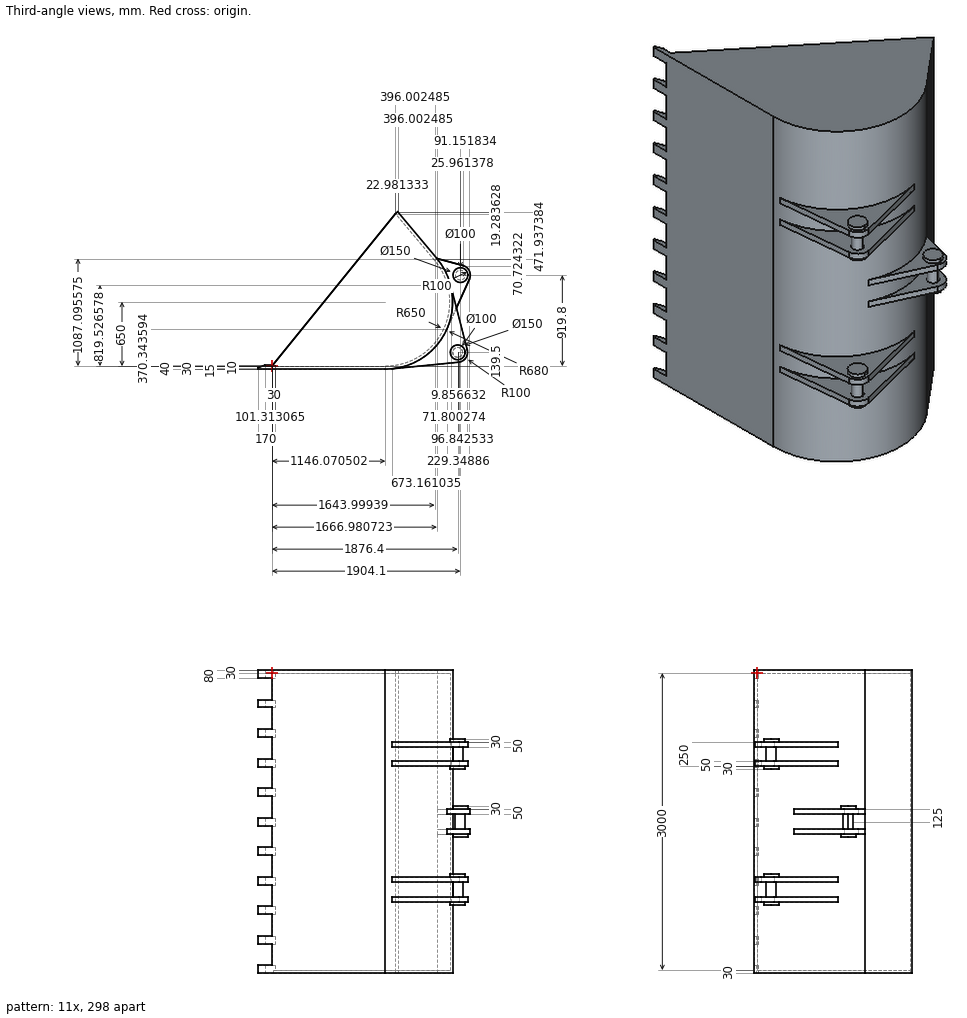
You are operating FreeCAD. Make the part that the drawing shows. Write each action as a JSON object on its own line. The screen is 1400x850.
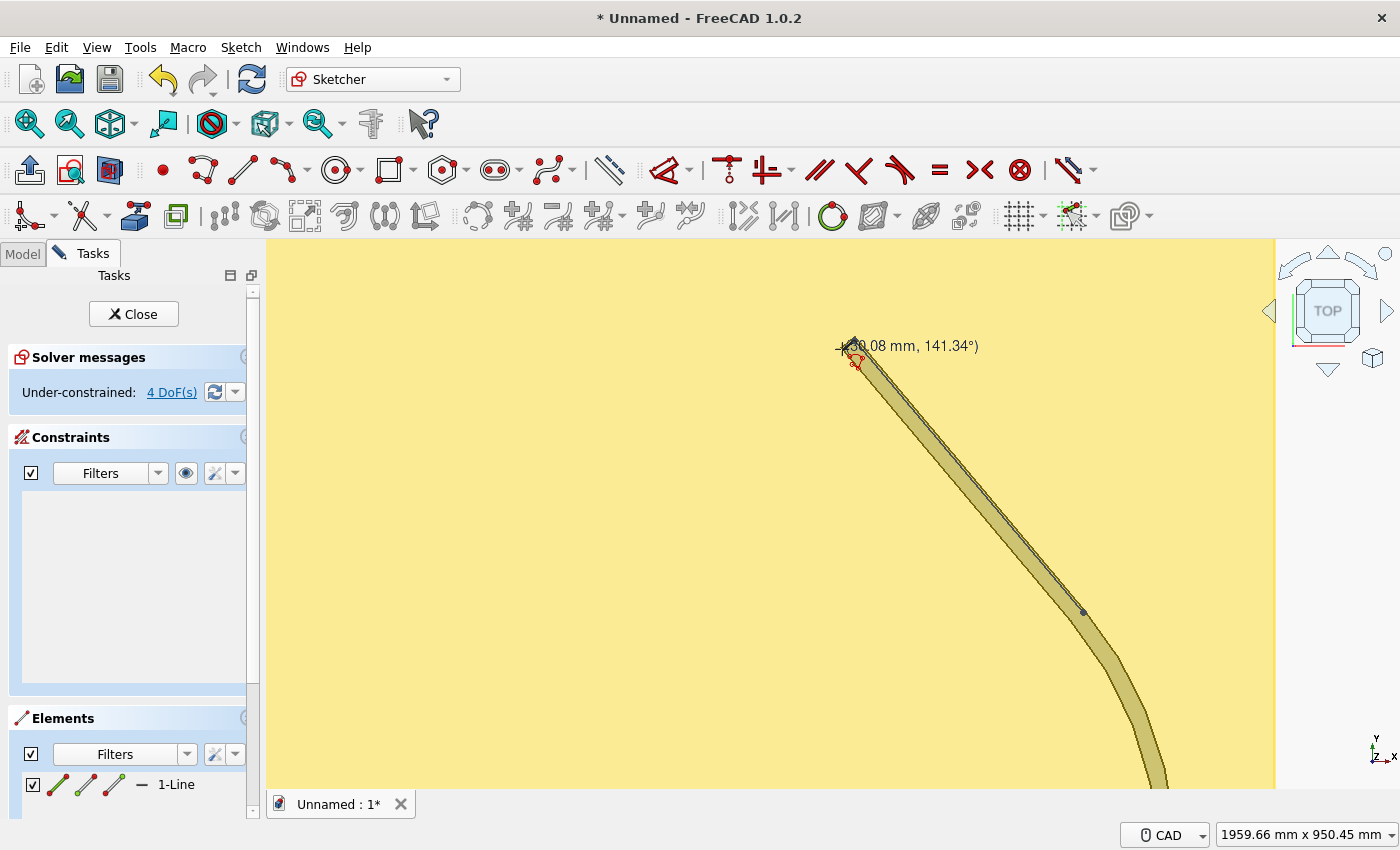
{"action": "left_click", "coordinate": [842, 348]}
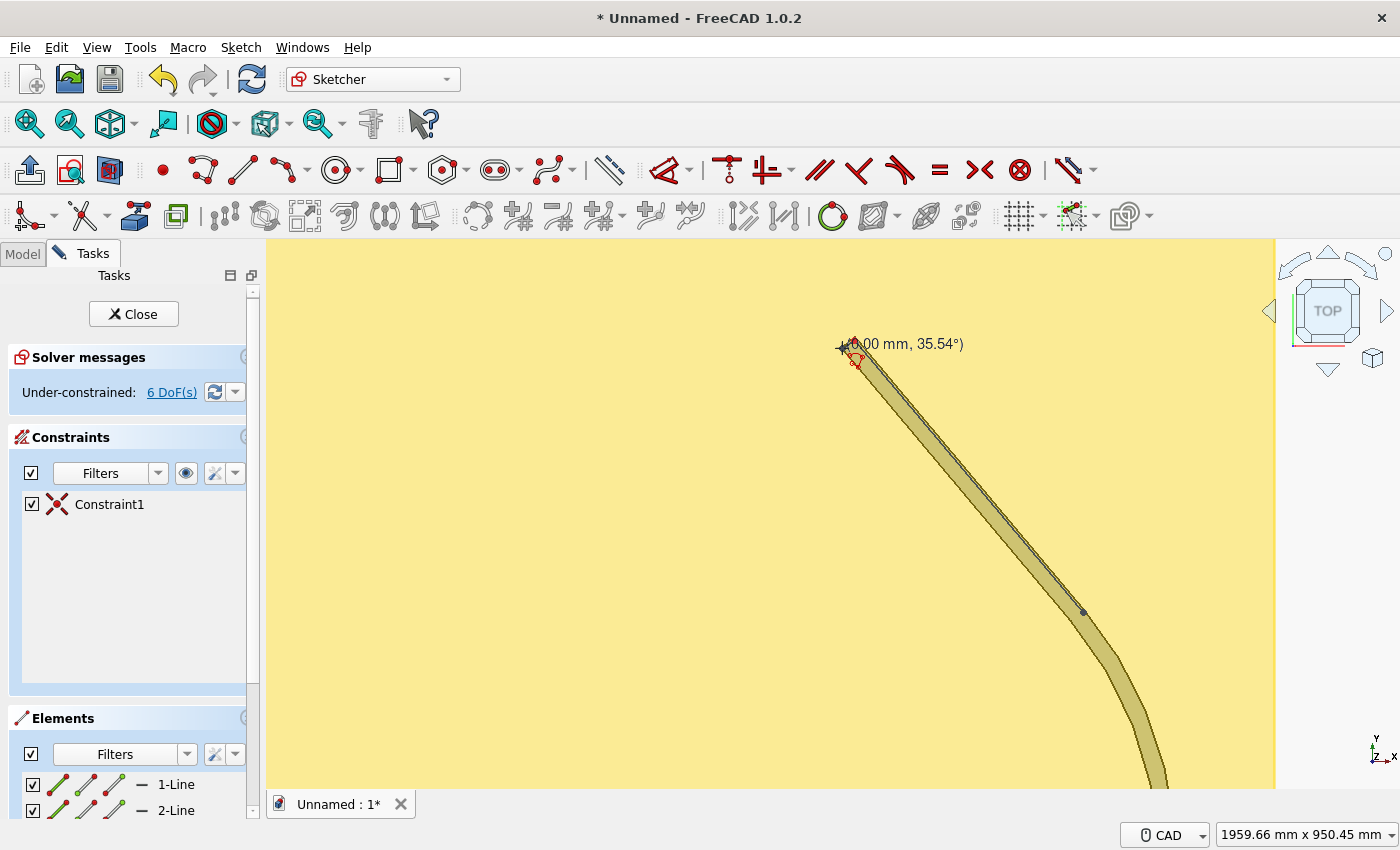
{"action": "scroll", "coordinate": [843, 350], "scroll_direction": "down", "scroll_amount": 5}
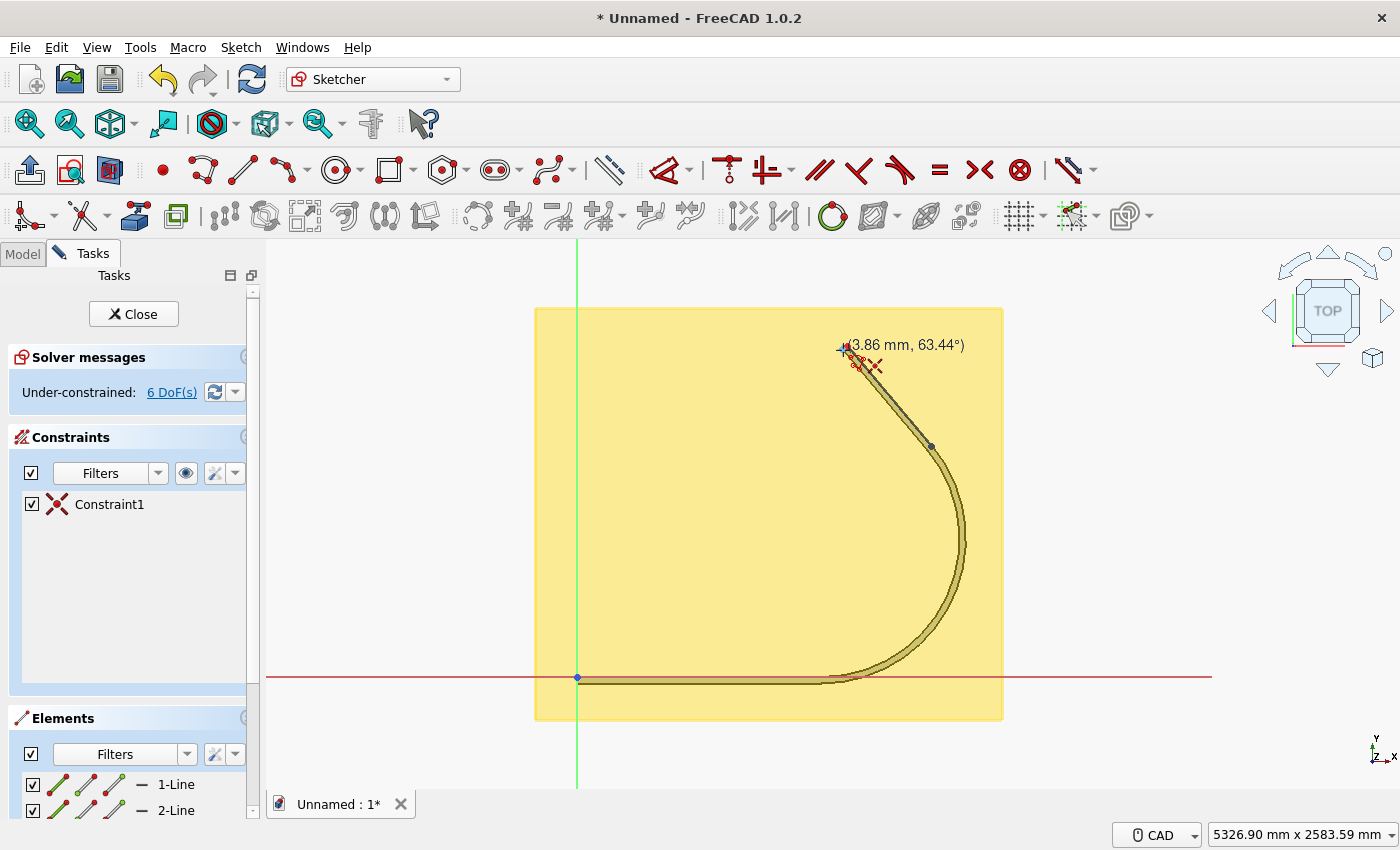
{"action": "left_click", "coordinate": [577, 677]}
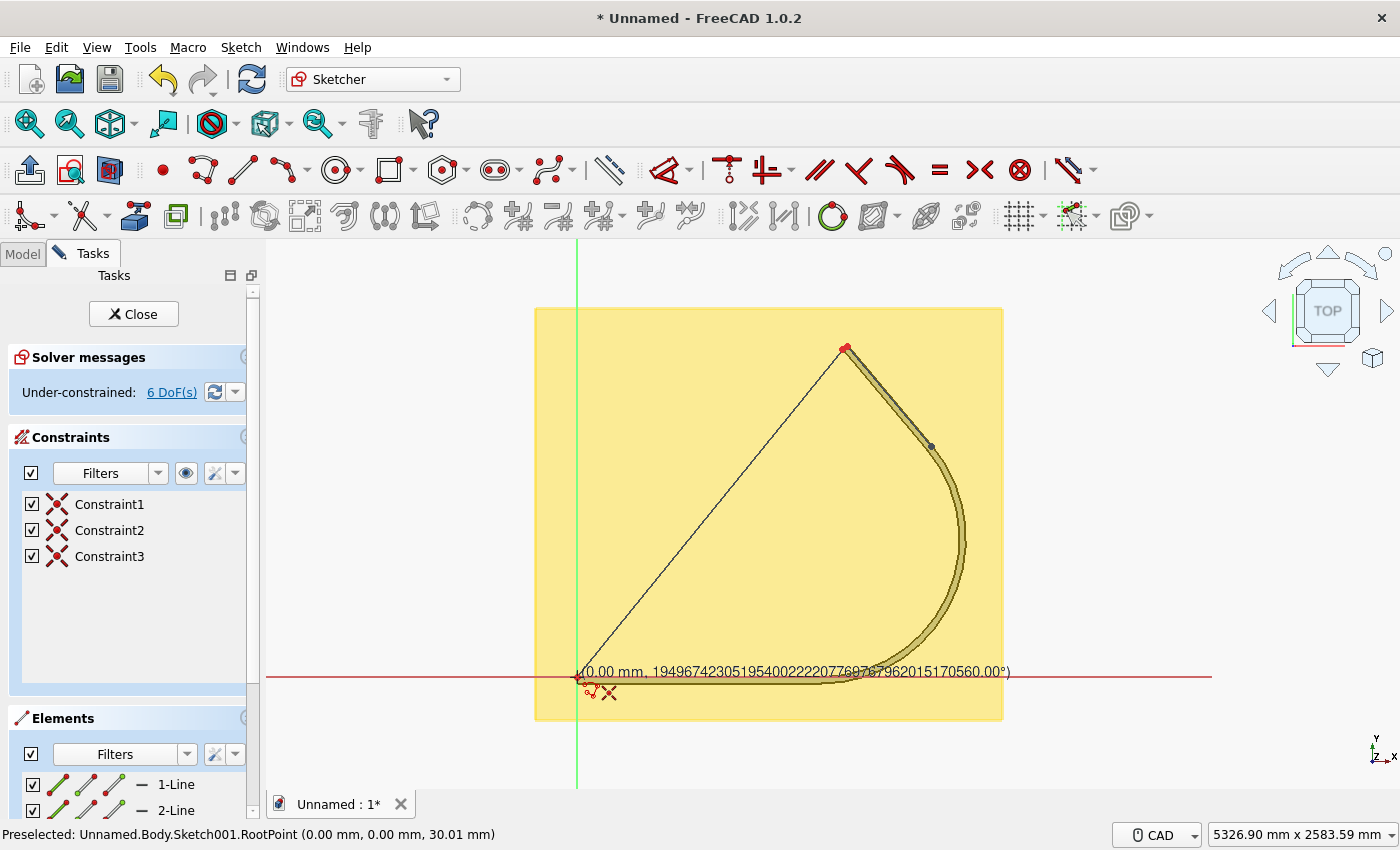
{"action": "scroll", "coordinate": [577, 684], "scroll_direction": "up", "scroll_amount": 5}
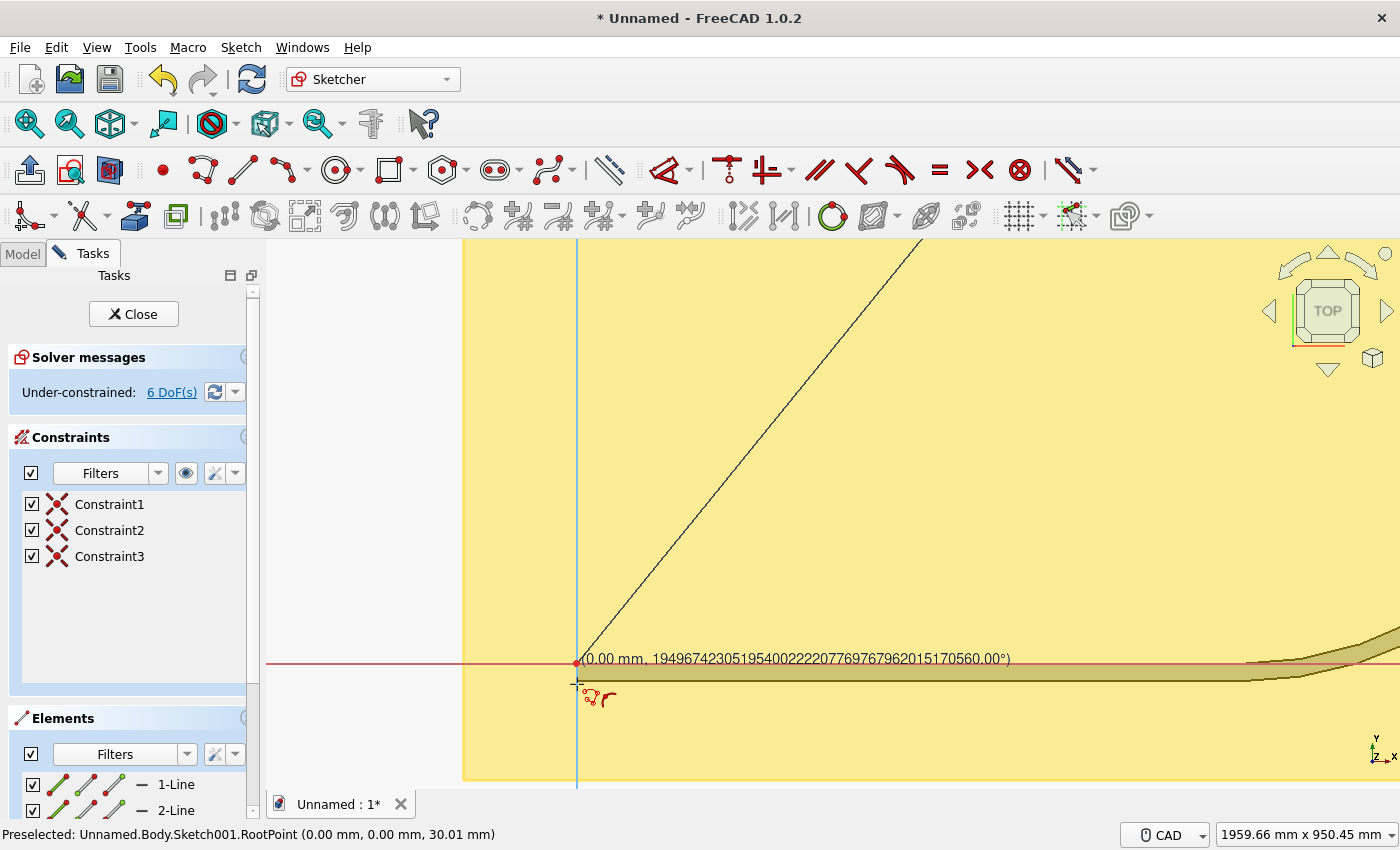
{"action": "left_click", "coordinate": [586, 681]}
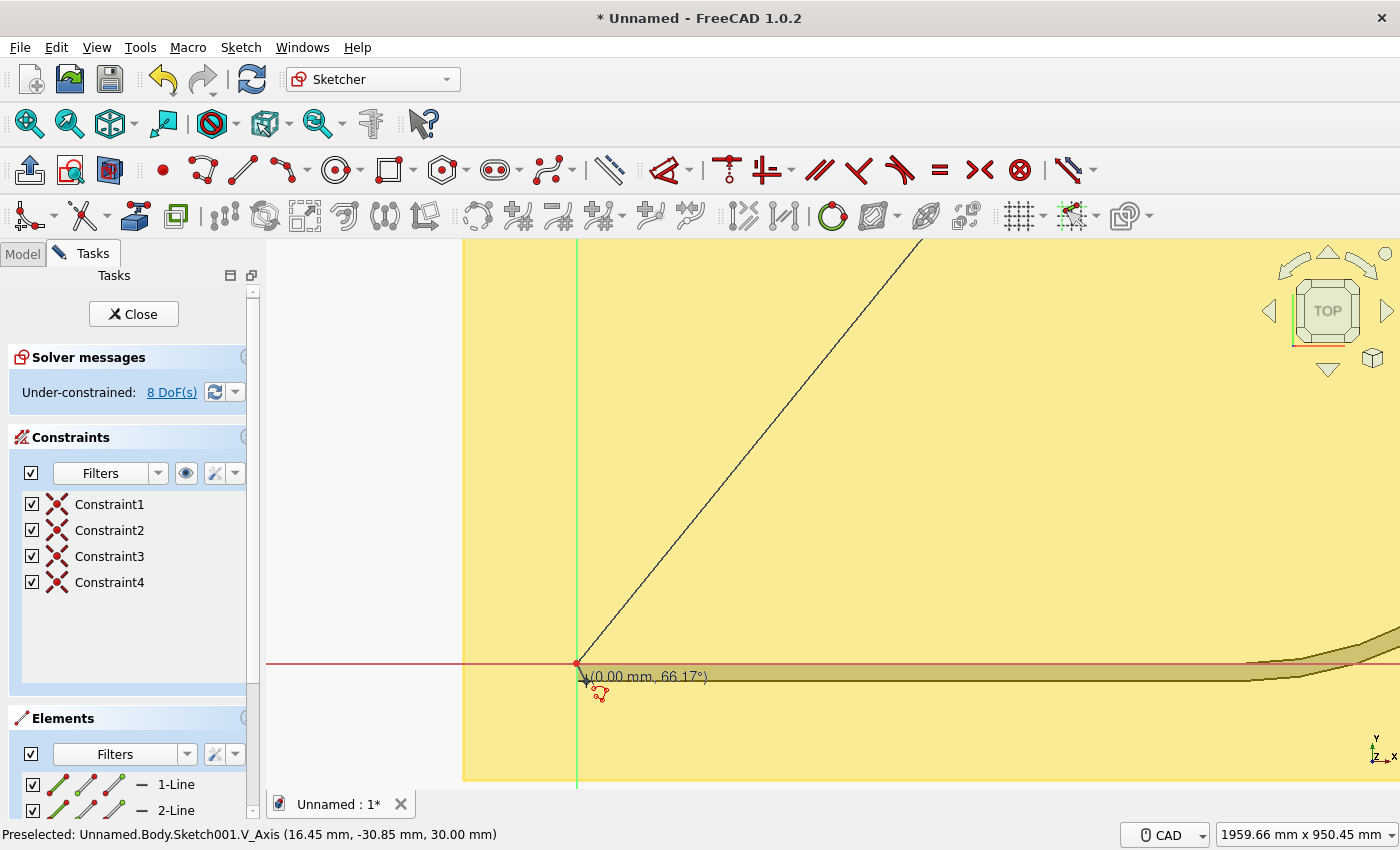
{"action": "scroll", "coordinate": [577, 684], "scroll_direction": "down", "scroll_amount": 5}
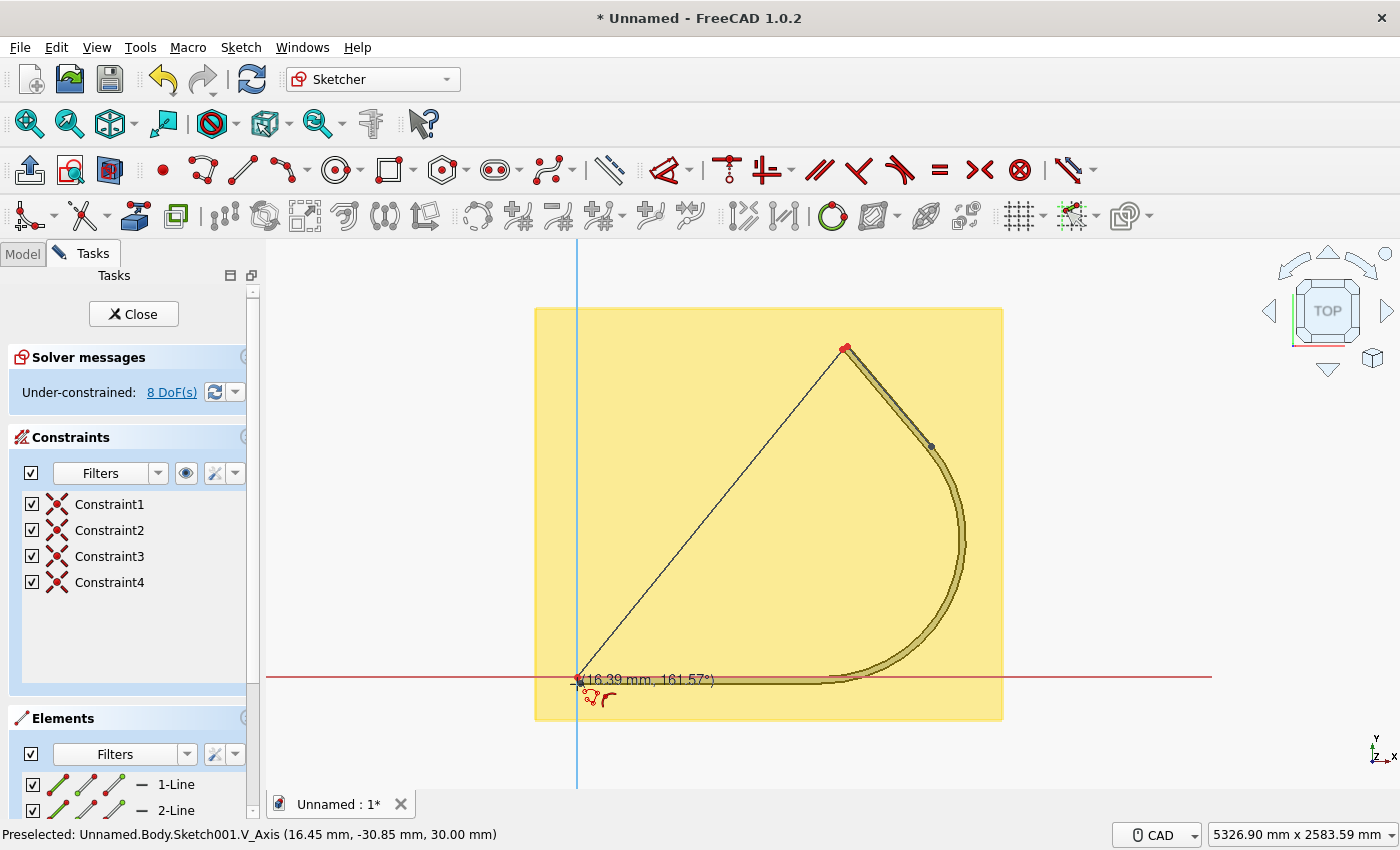
{"action": "scroll", "coordinate": [821, 684], "scroll_direction": "up", "scroll_amount": 5}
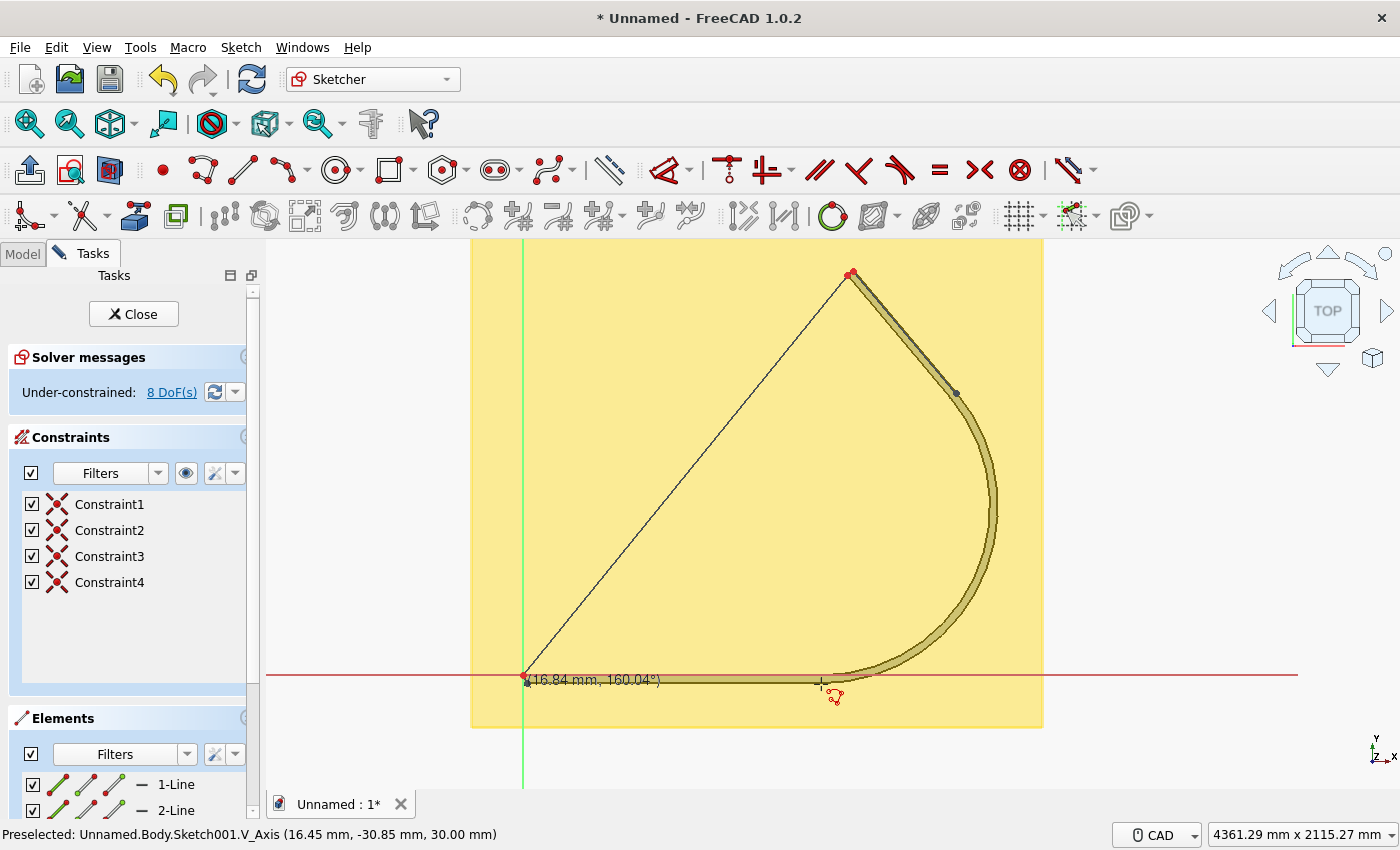
{"action": "left_click", "coordinate": [820, 681]}
{"action": "right_click", "coordinate": [820, 681]}